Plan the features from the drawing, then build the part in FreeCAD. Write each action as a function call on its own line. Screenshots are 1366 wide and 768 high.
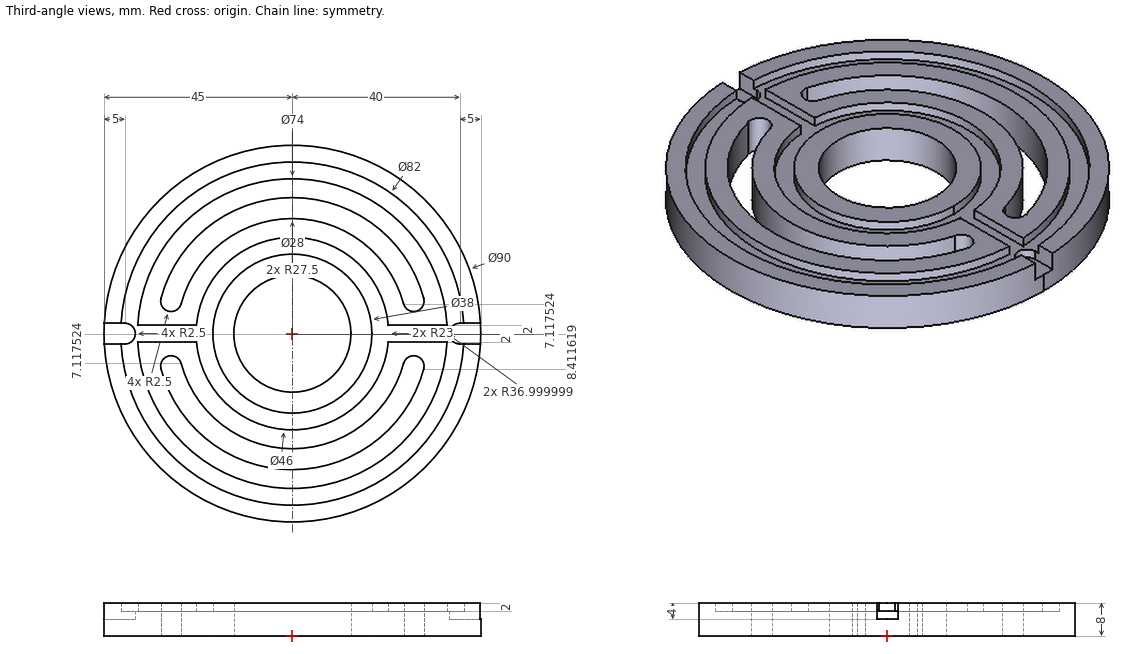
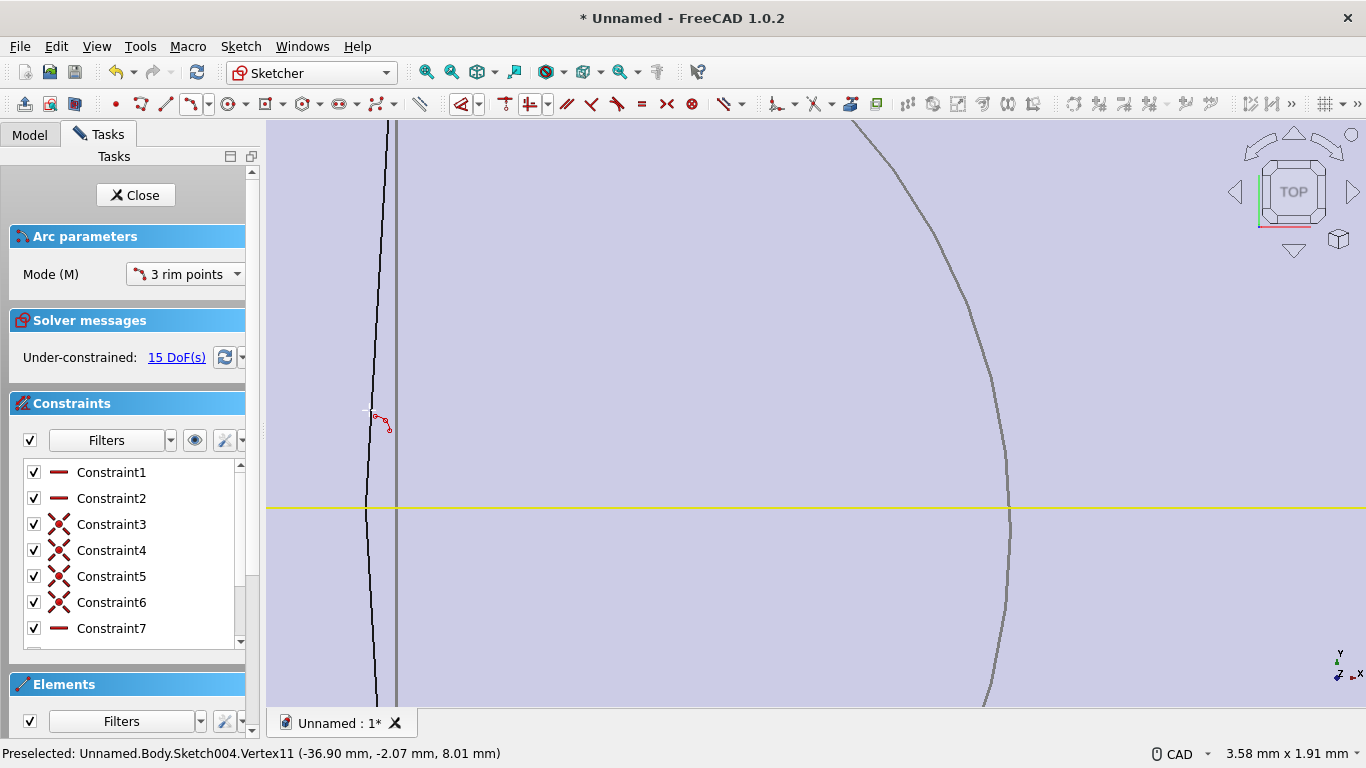
click(366, 386)
key(Escape)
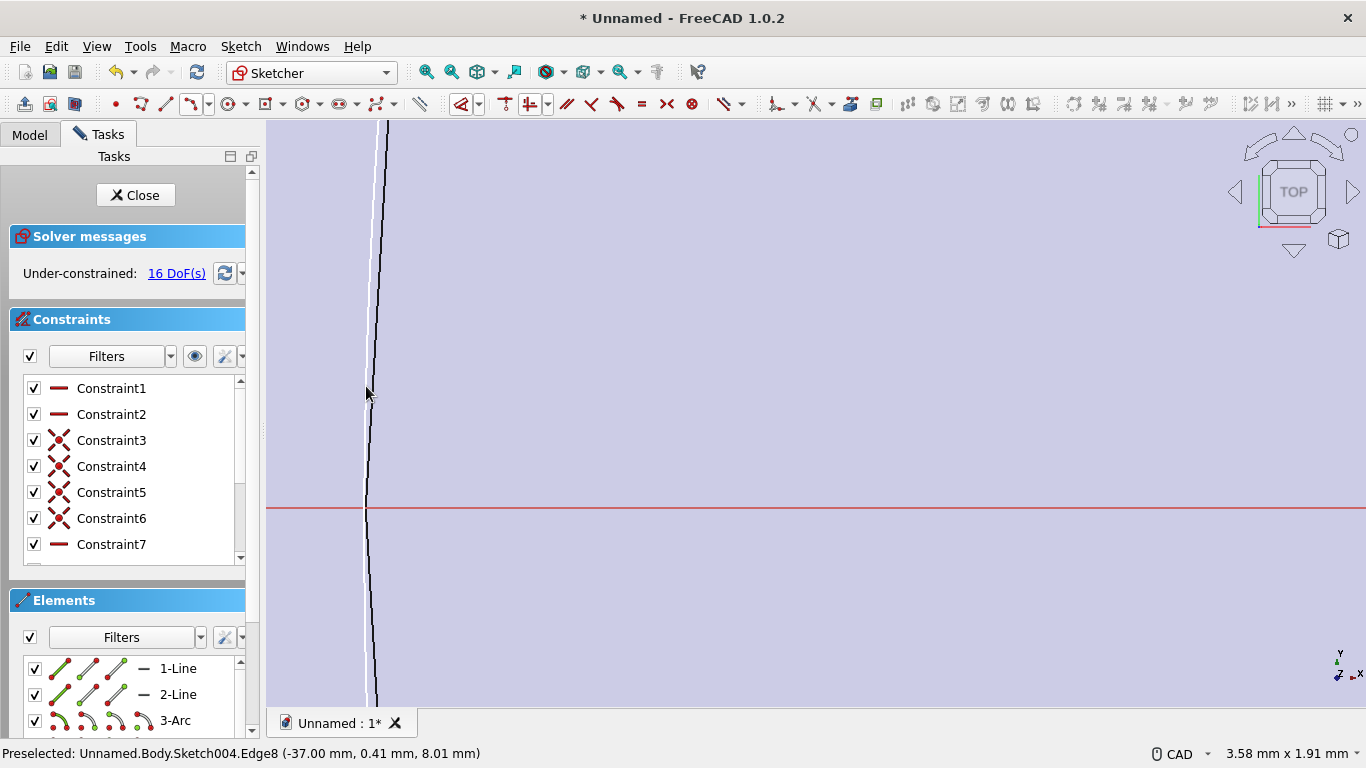
scroll(369, 410, down, 17)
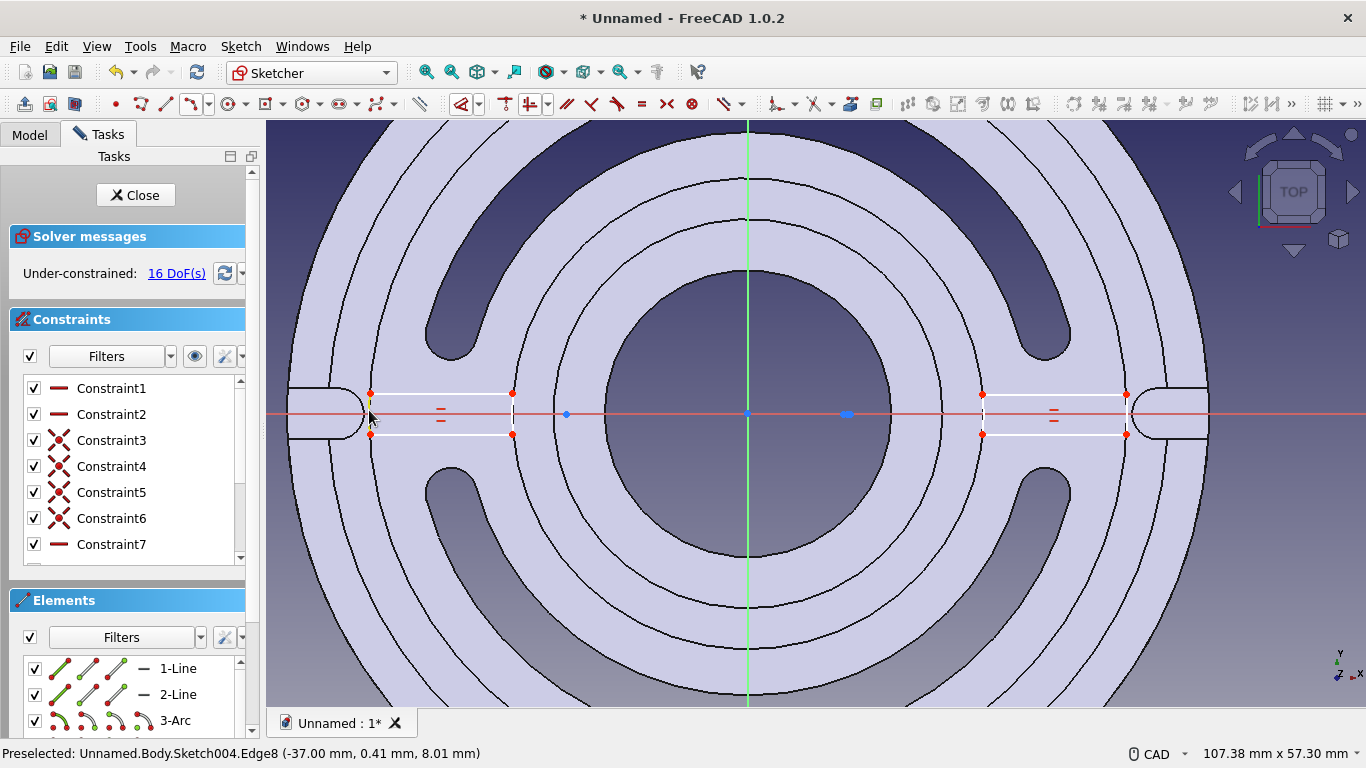
scroll(1127, 423, up, 3)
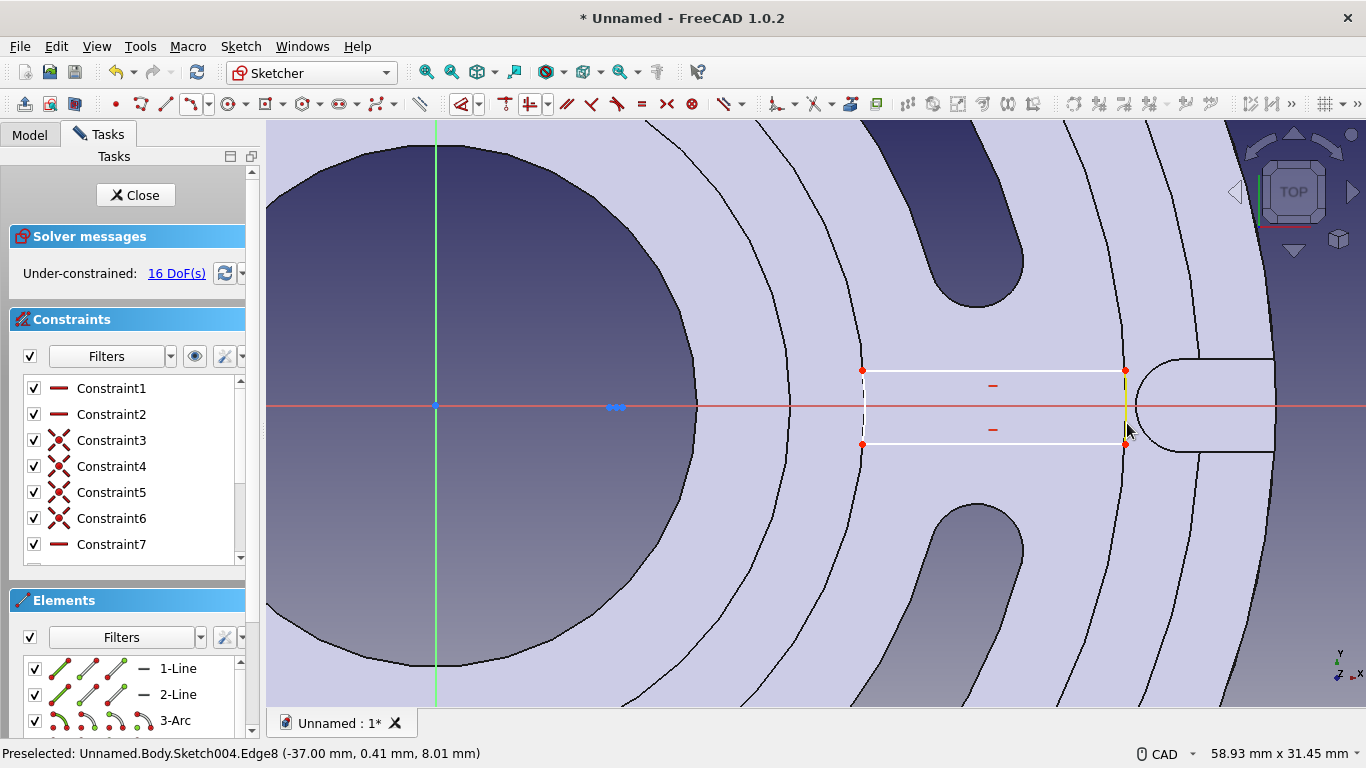
click(1126, 422)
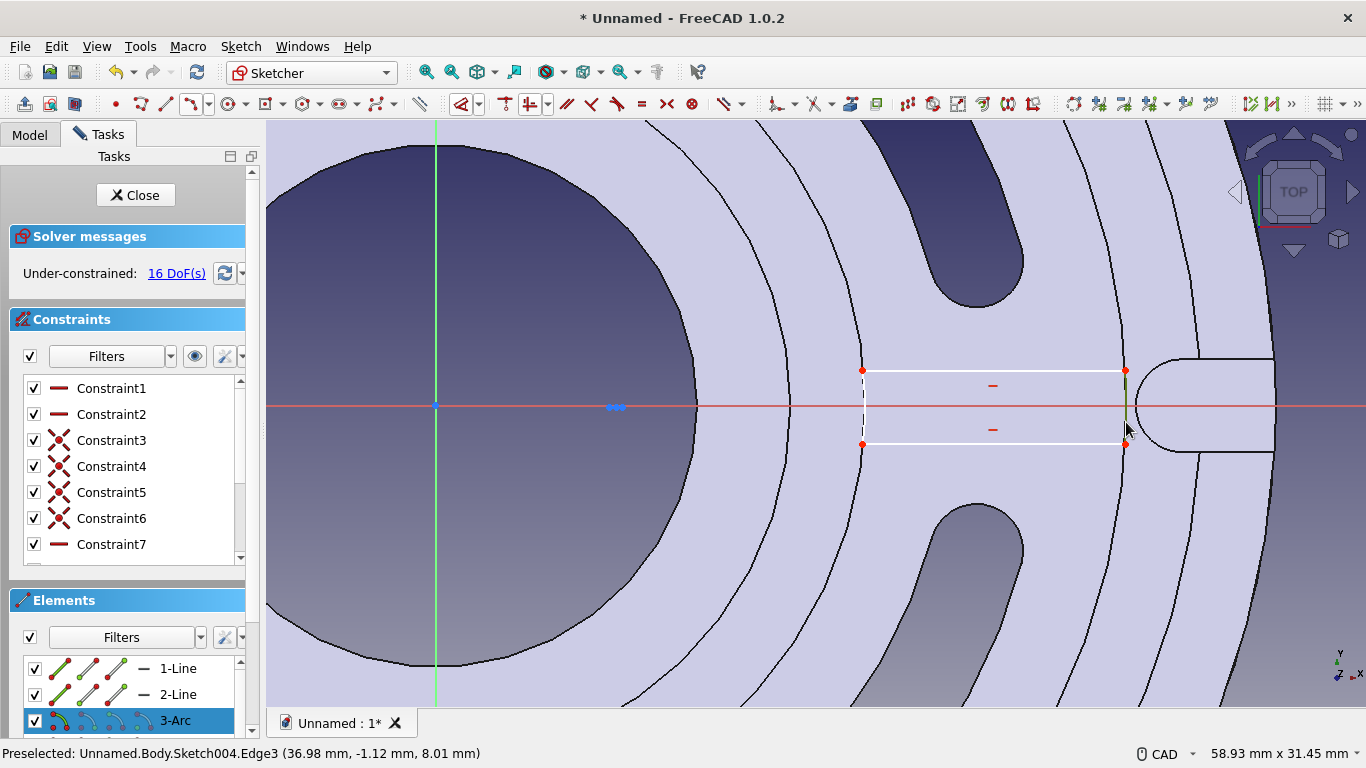
click(865, 422)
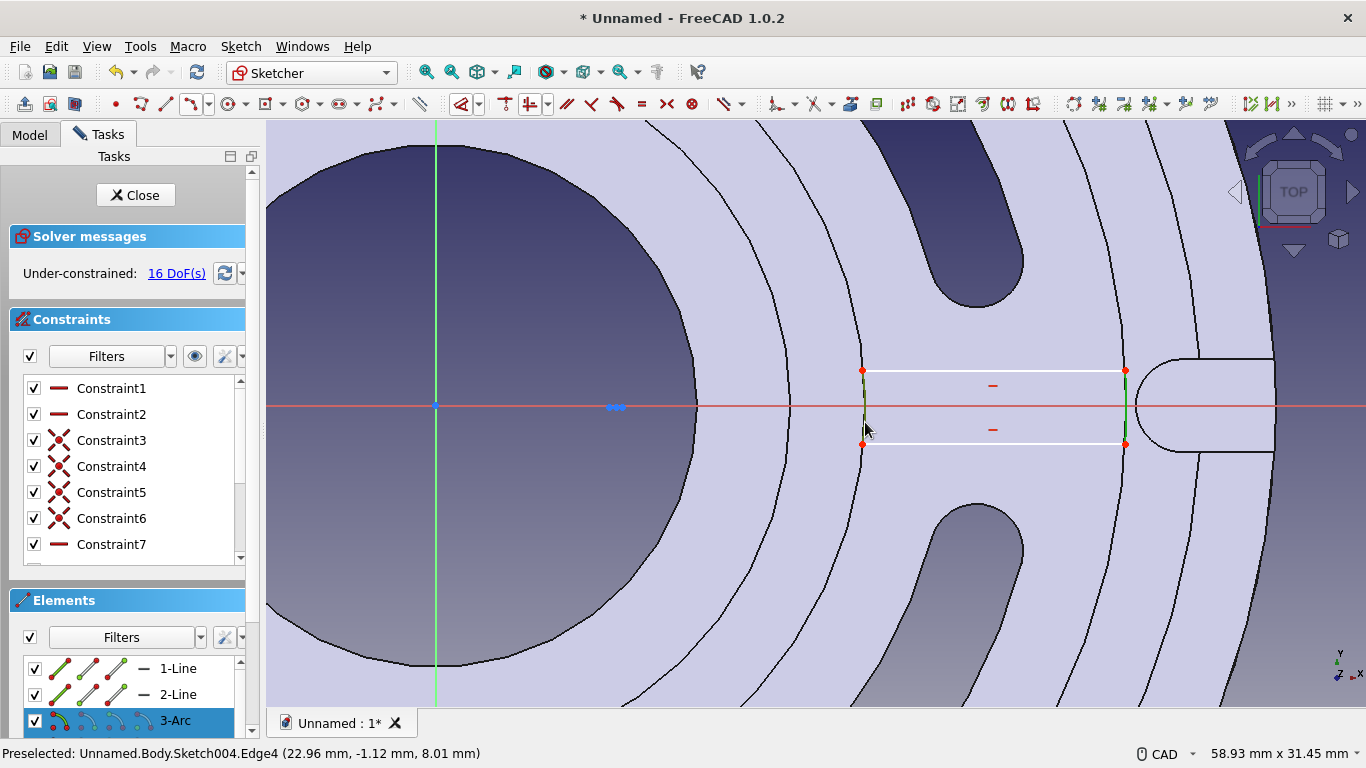
key(c)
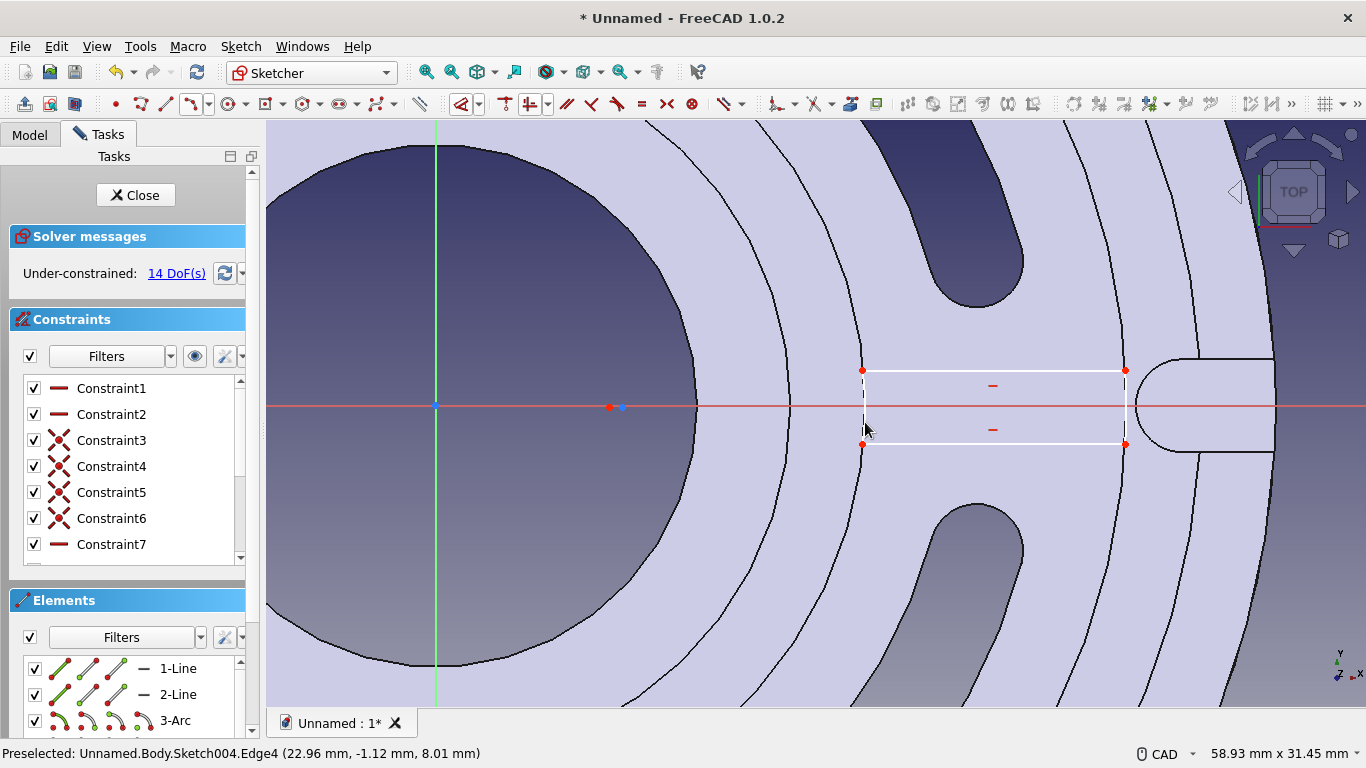
click(1126, 422)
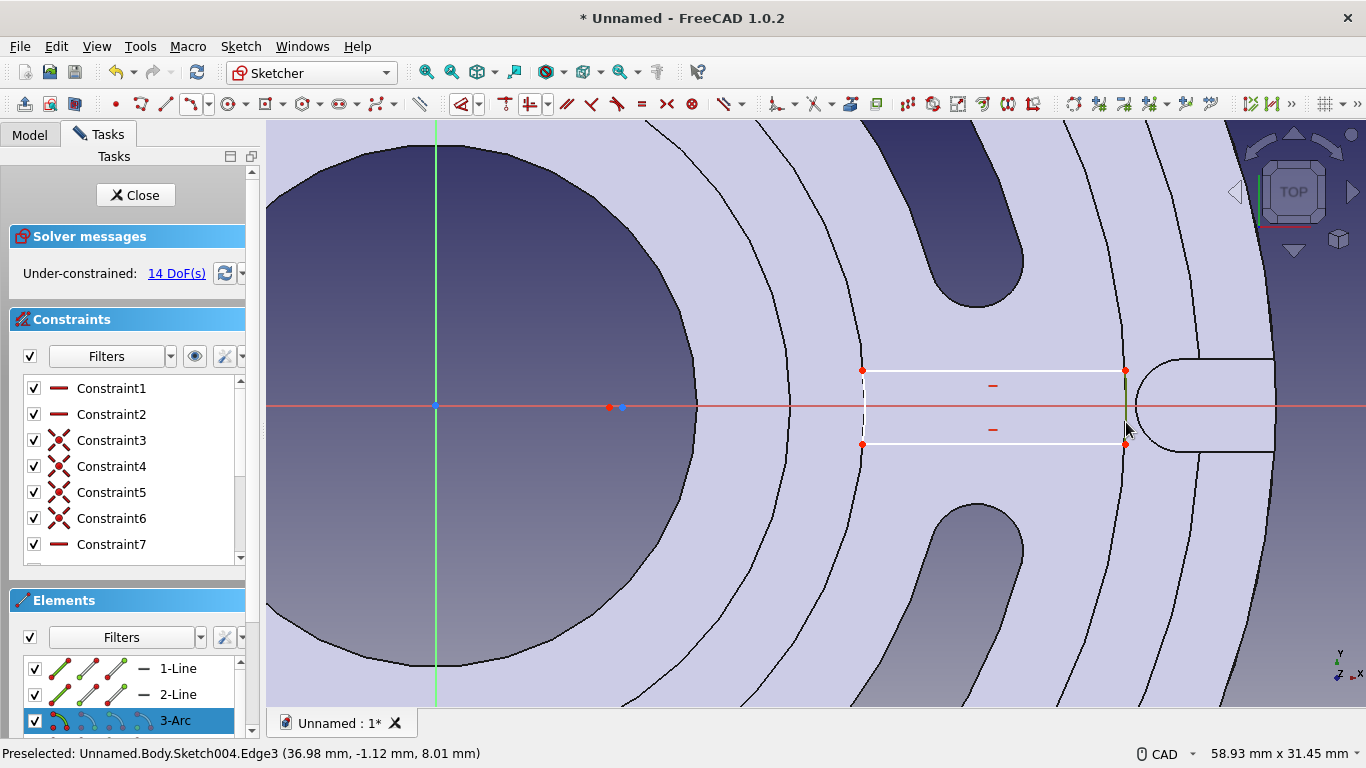
scroll(1002, 420, down, 4)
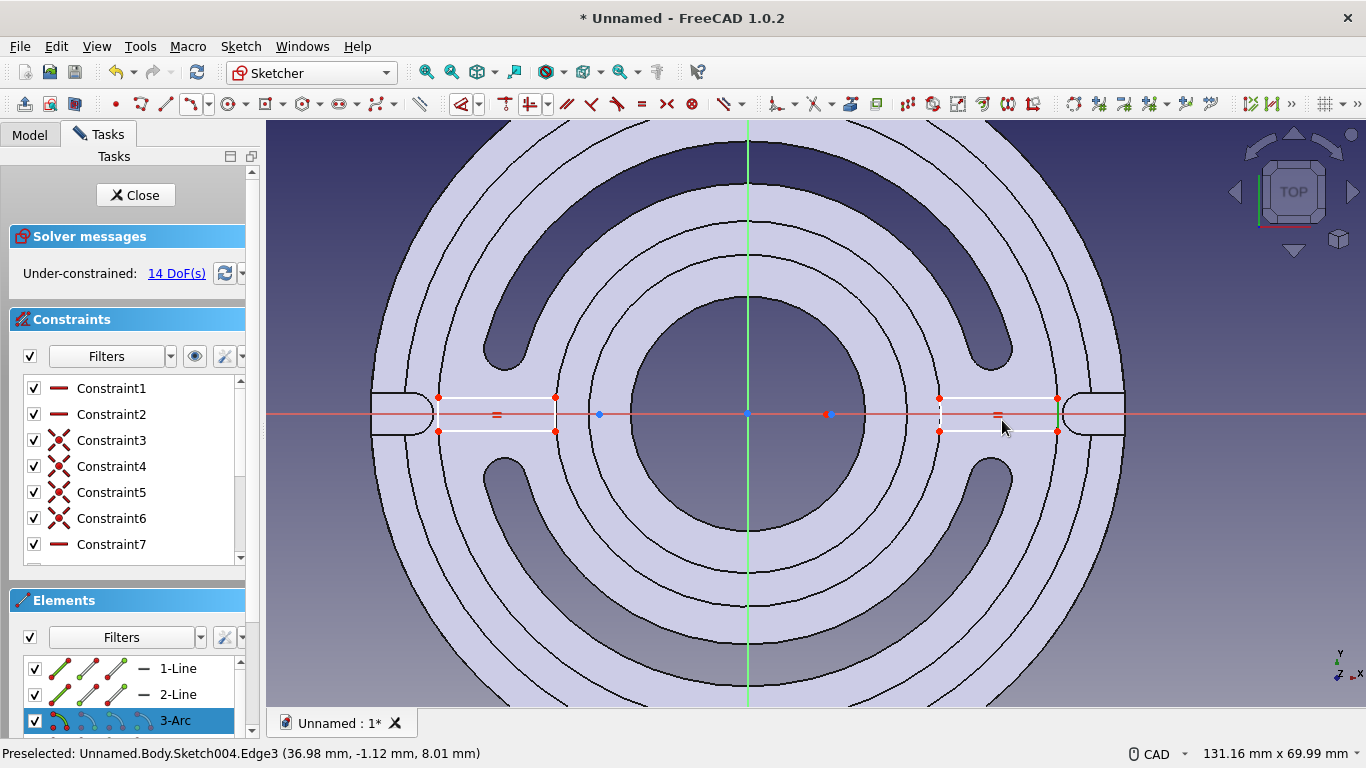
scroll(555, 408, up, 5)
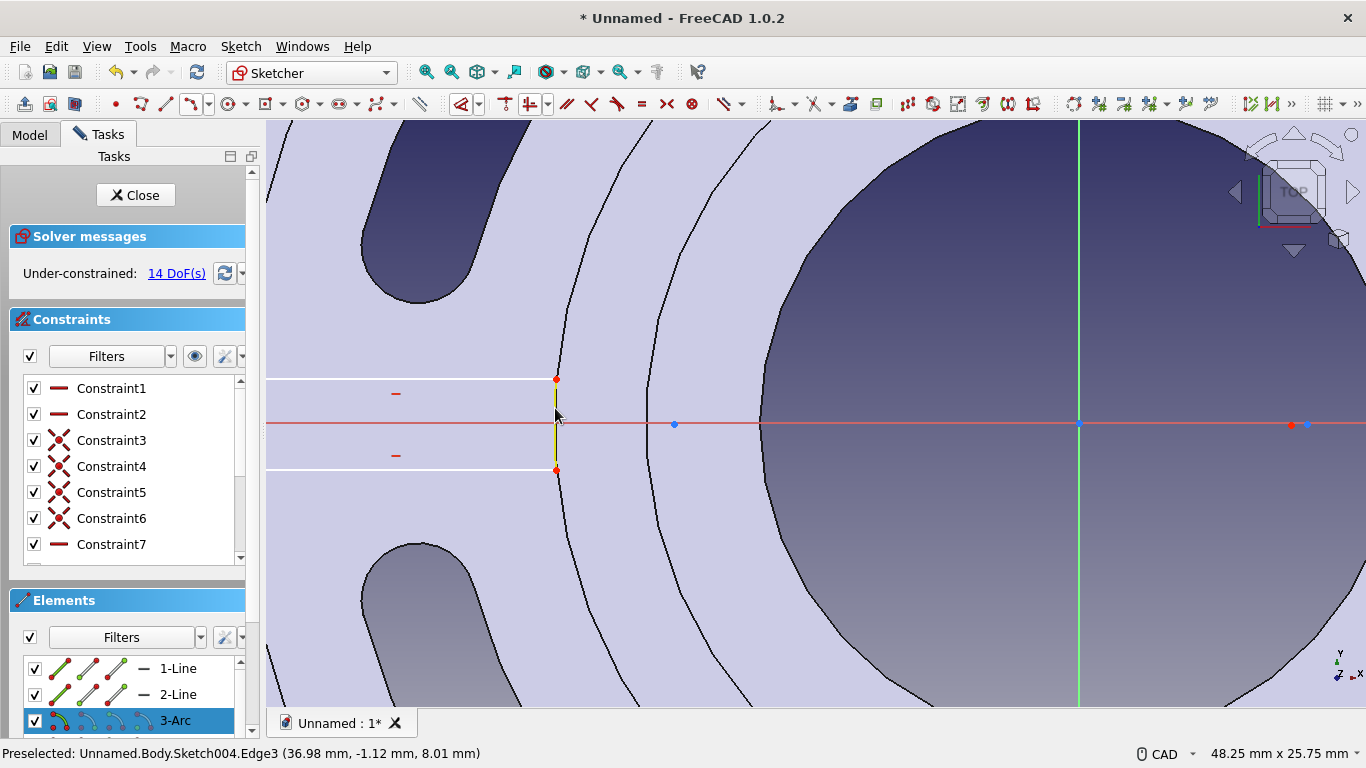
click(555, 407)